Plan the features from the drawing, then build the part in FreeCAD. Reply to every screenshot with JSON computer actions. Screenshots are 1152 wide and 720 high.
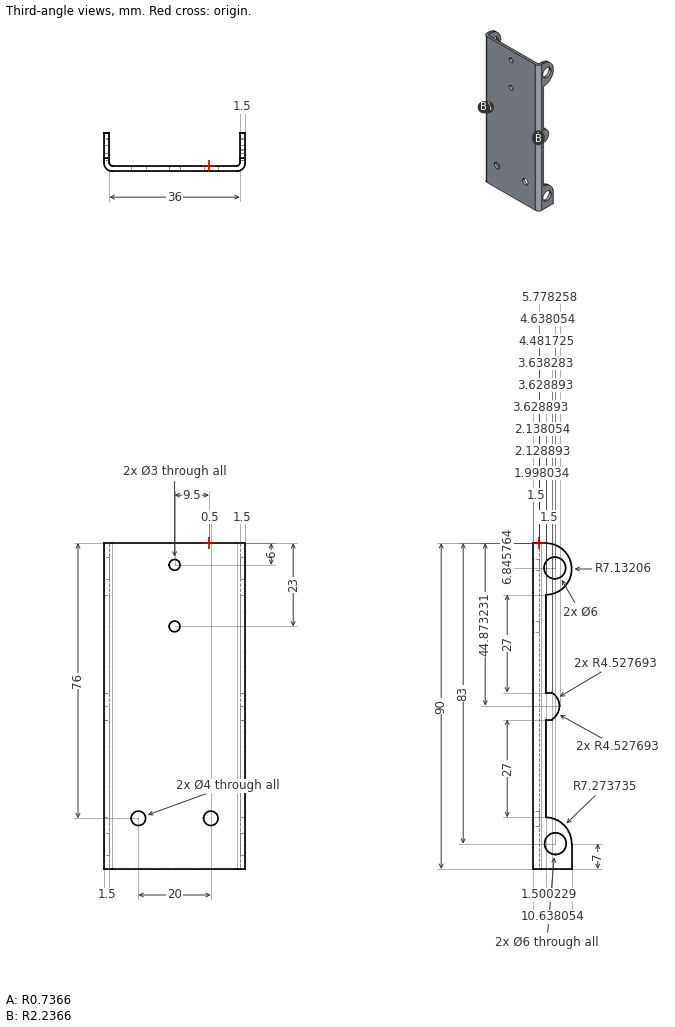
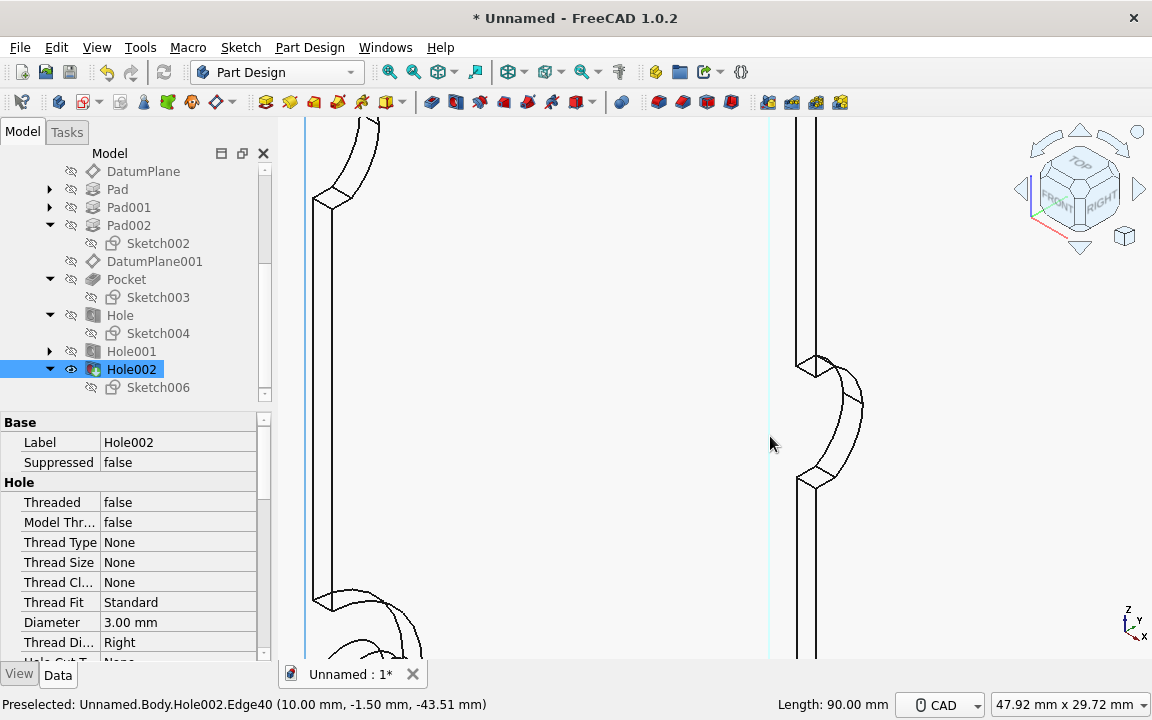
{"action": "left_click", "coordinate": [390, 72]}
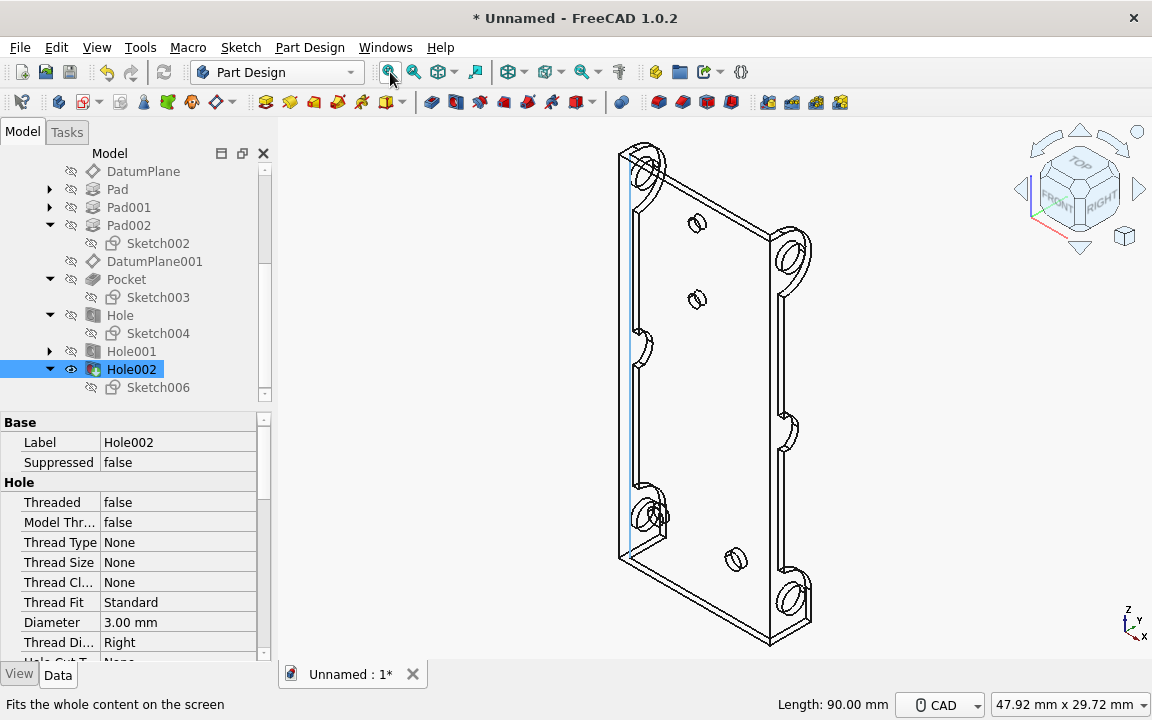
{"action": "key", "text": "2"}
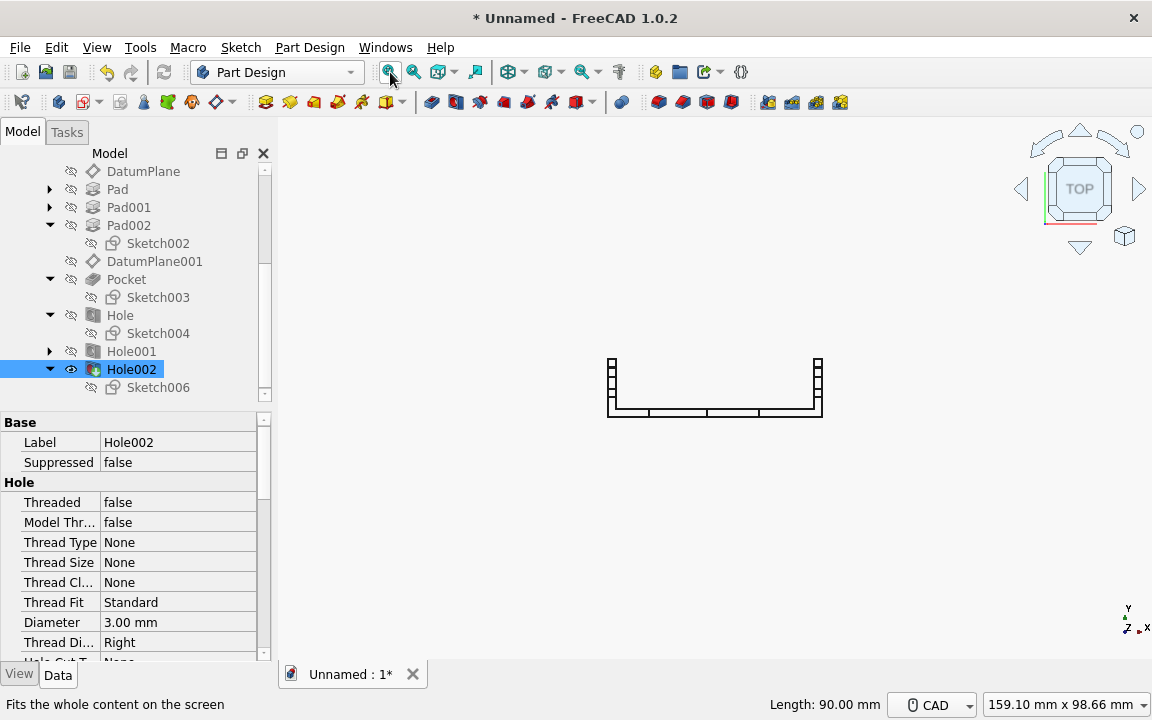
{"action": "left_click", "coordinate": [390, 72]}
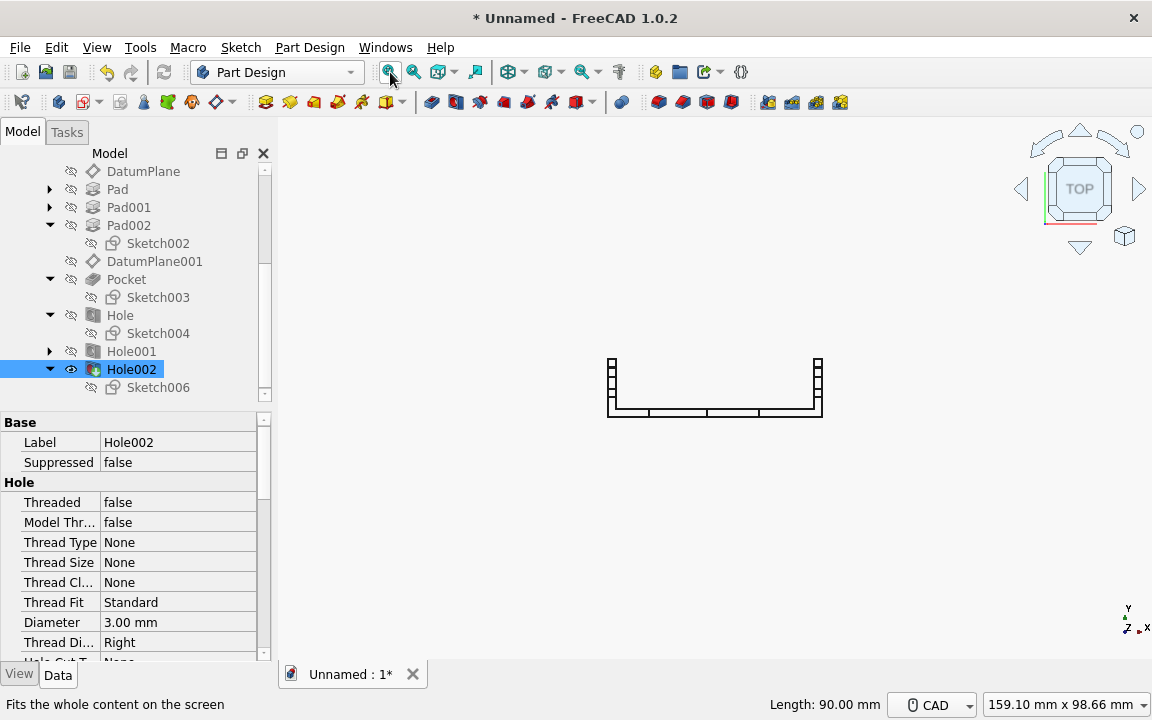
{"action": "scroll", "coordinate": [814, 408], "scroll_direction": "up", "scroll_amount": 6}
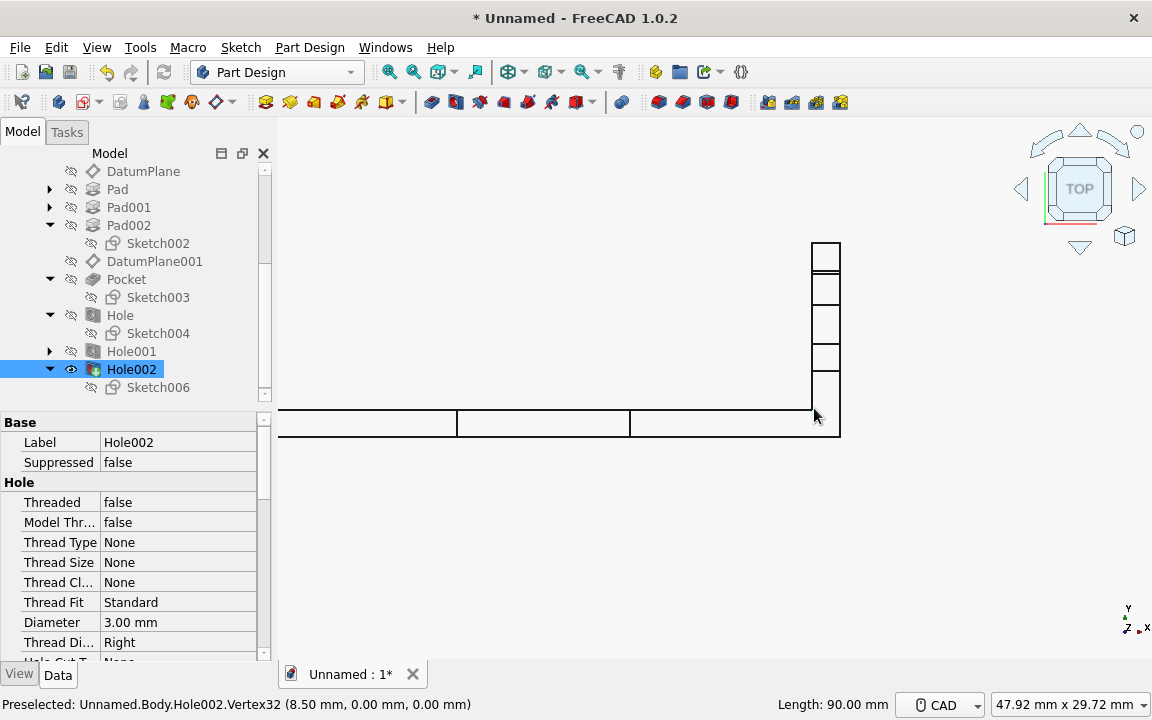
{"action": "left_click", "coordinate": [390, 72]}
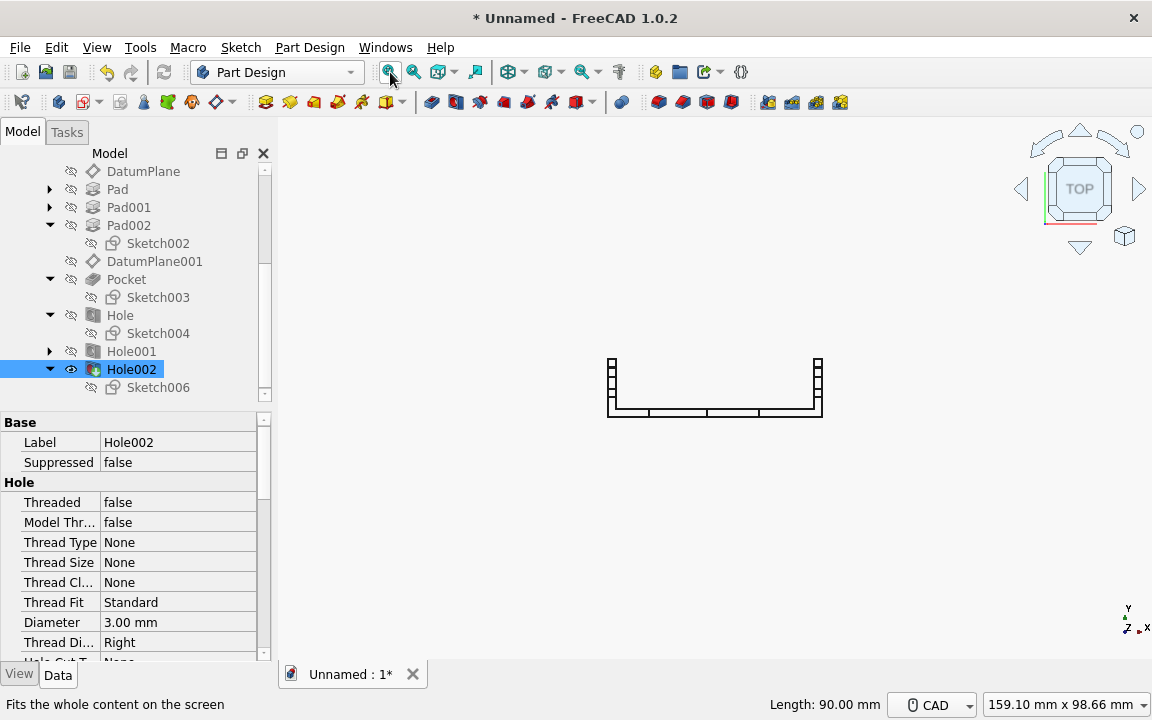
{"action": "key", "text": "1"}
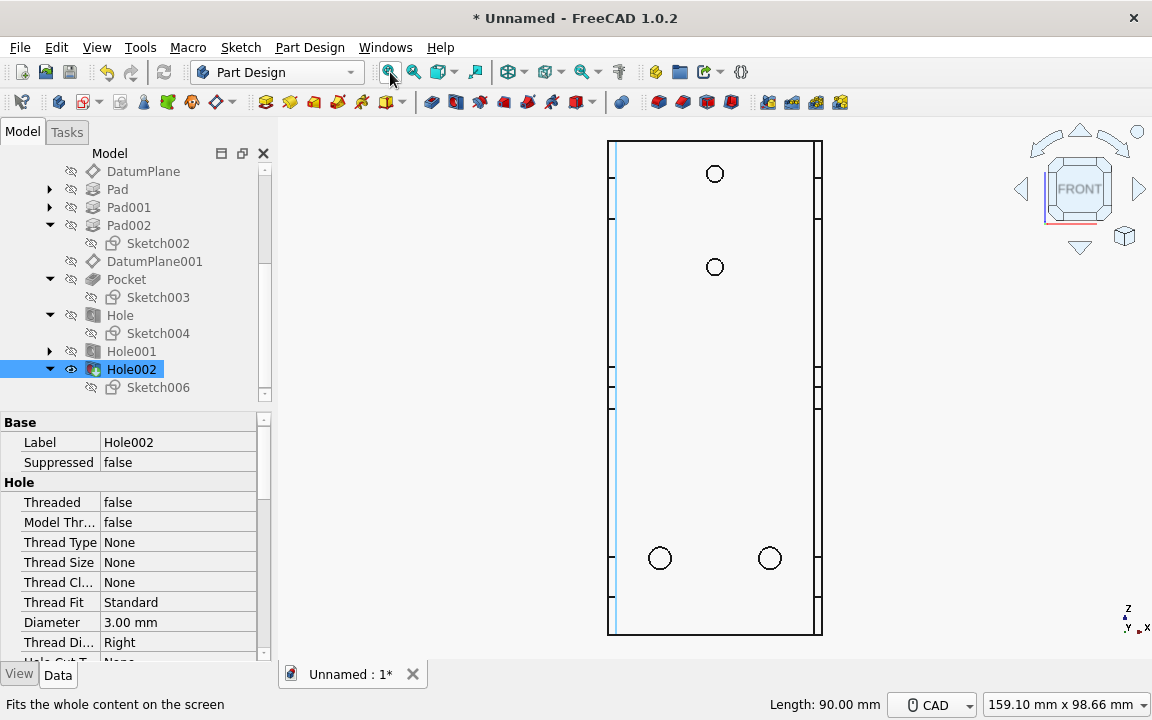
{"action": "left_click", "coordinate": [814, 387], "text": "ctrl"}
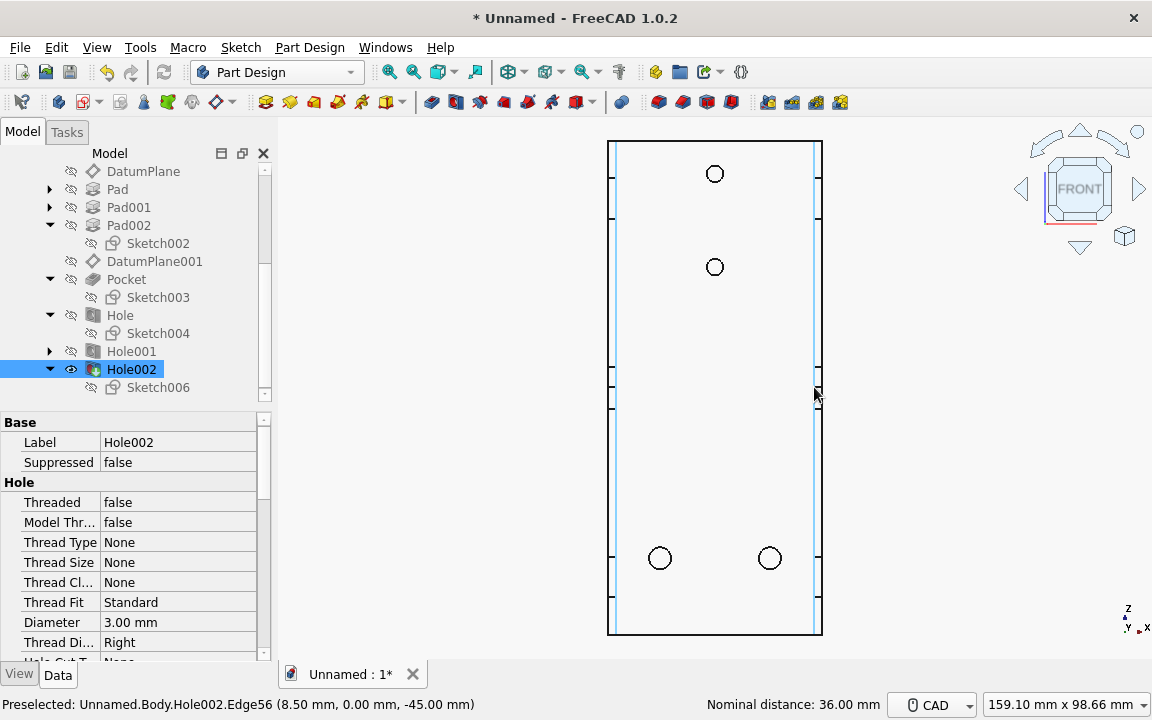
{"action": "key", "text": "v 1"}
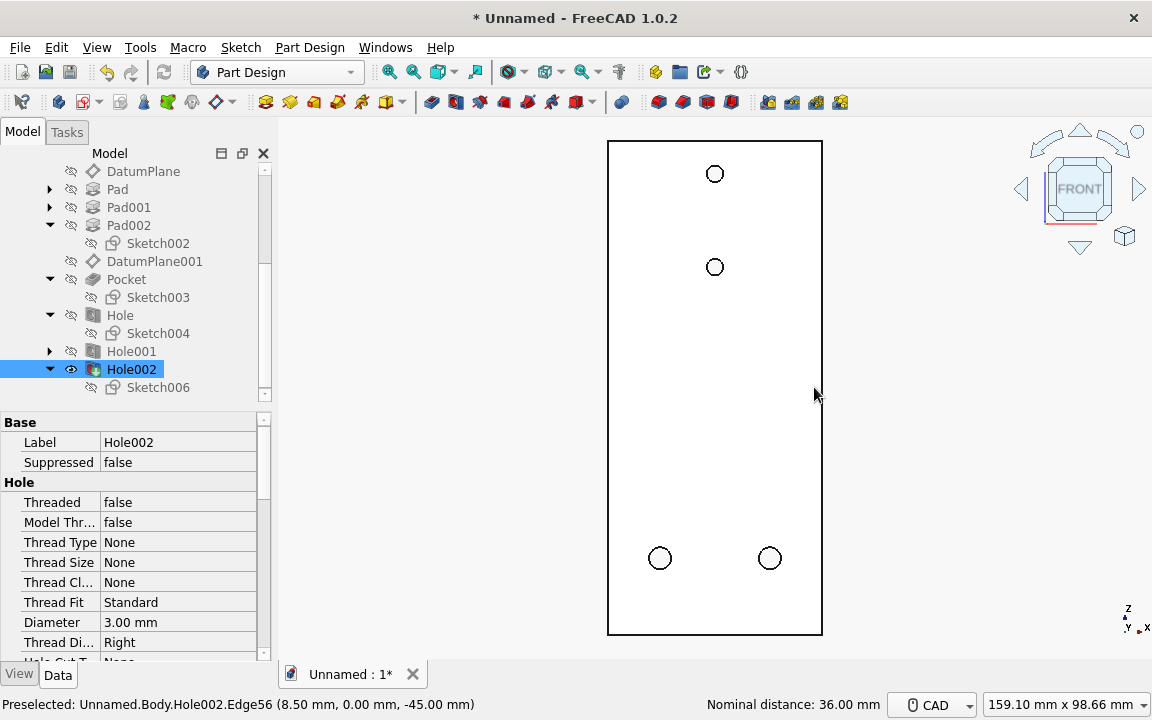
{"action": "left_click", "coordinate": [660, 102]}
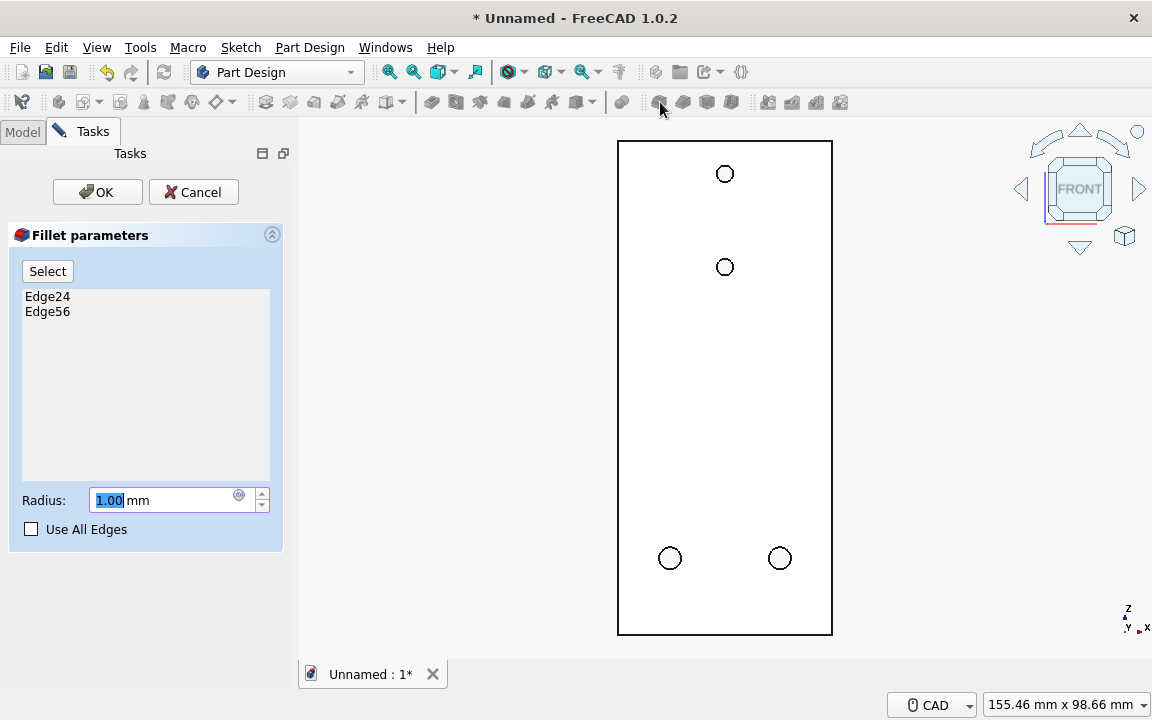
{"action": "type", "text": "0.7366"}
{"action": "key", "text": "Tab"}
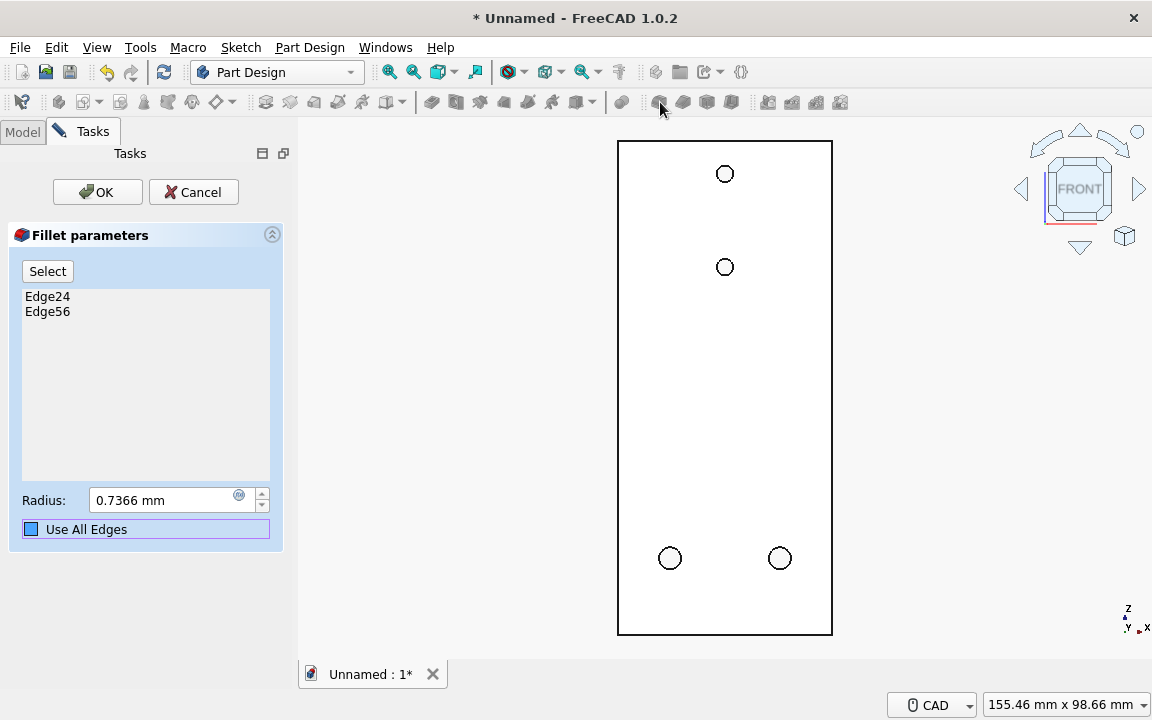
{"action": "left_click", "coordinate": [98, 192]}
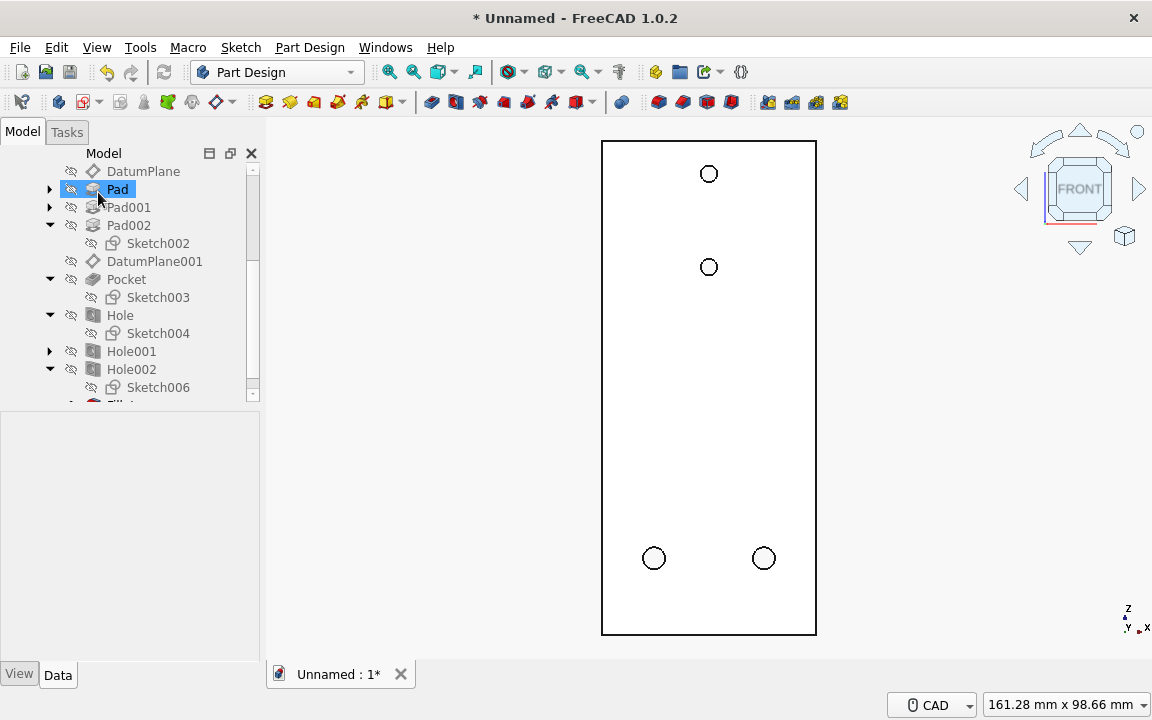
{"action": "left_click", "coordinate": [602, 387]}